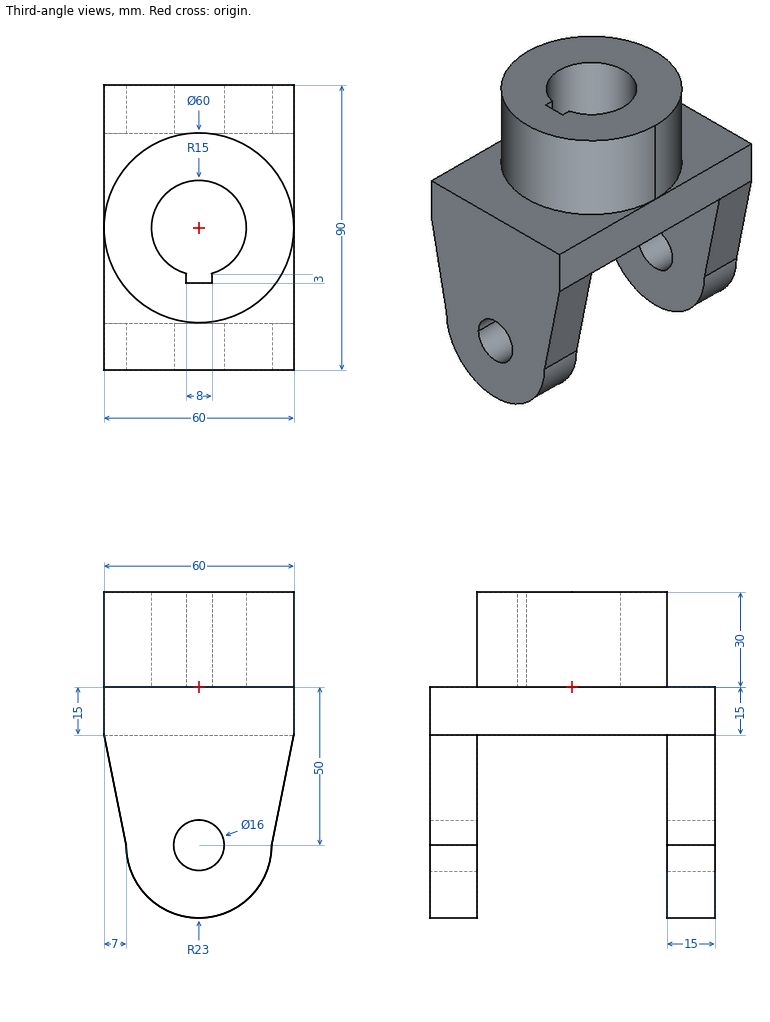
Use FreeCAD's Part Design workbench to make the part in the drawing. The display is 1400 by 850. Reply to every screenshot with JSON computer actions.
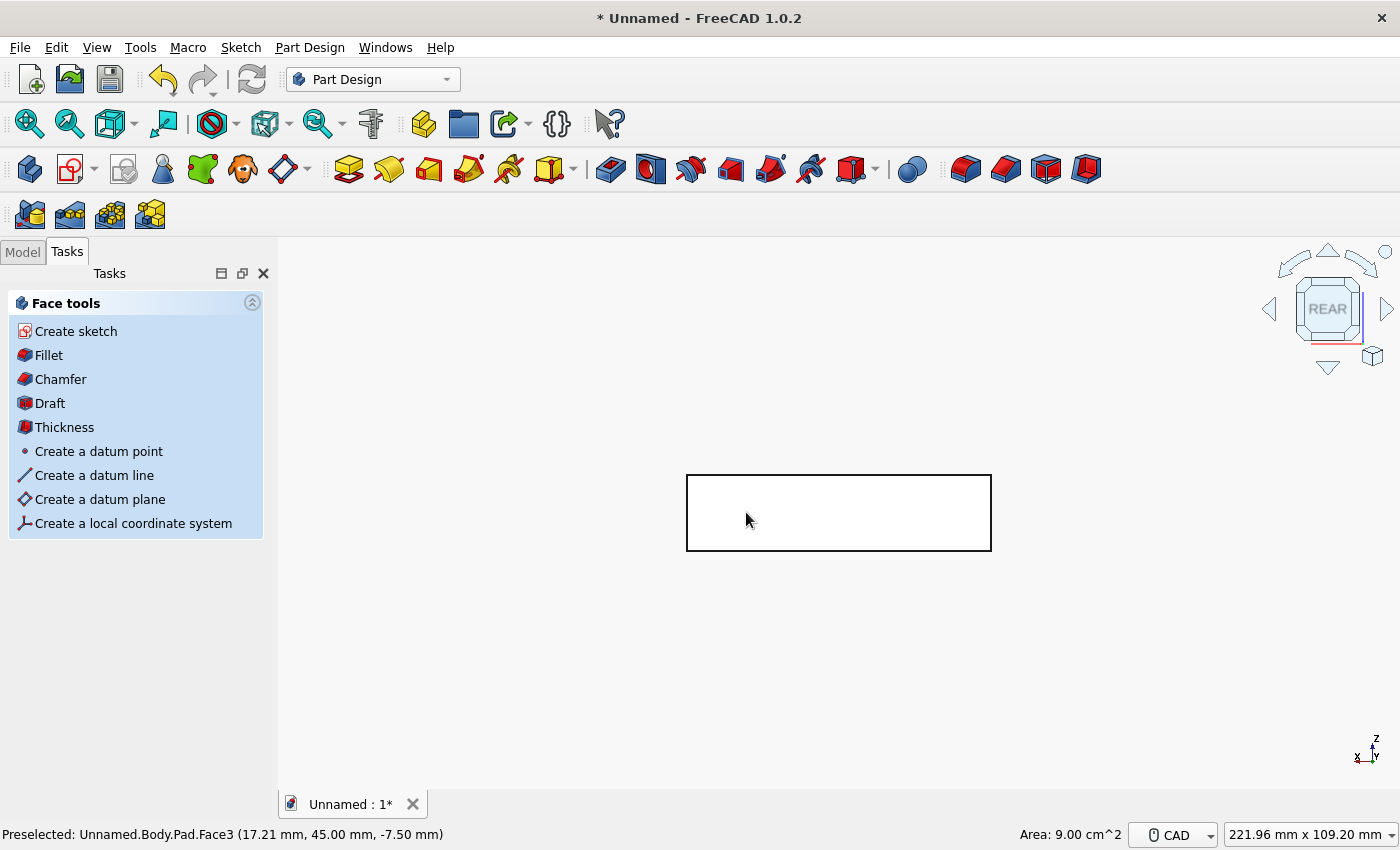
{"action": "left_click", "coordinate": [70, 170]}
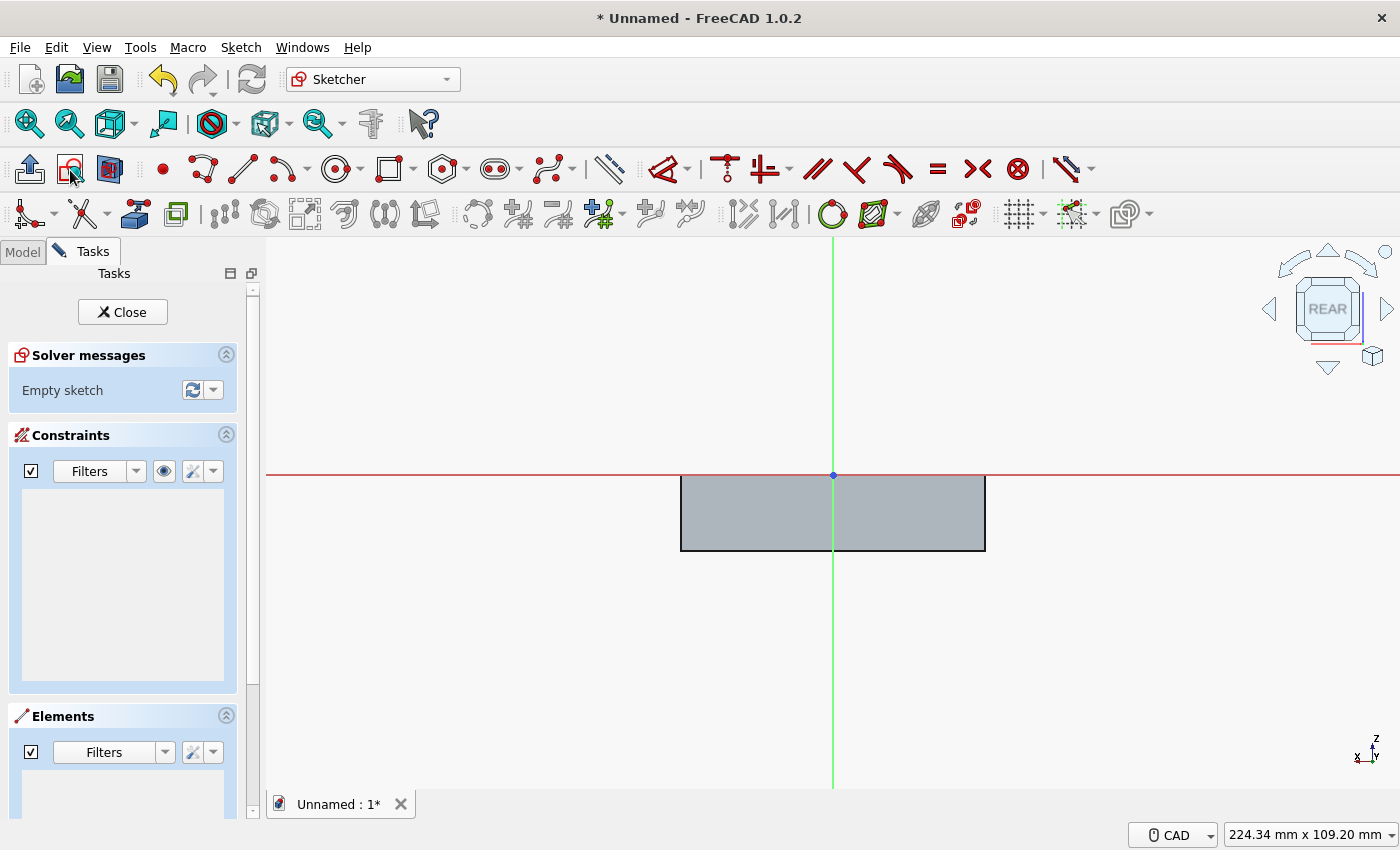
{"action": "scroll", "coordinate": [625, 265], "scroll_direction": "down", "scroll_amount": 2}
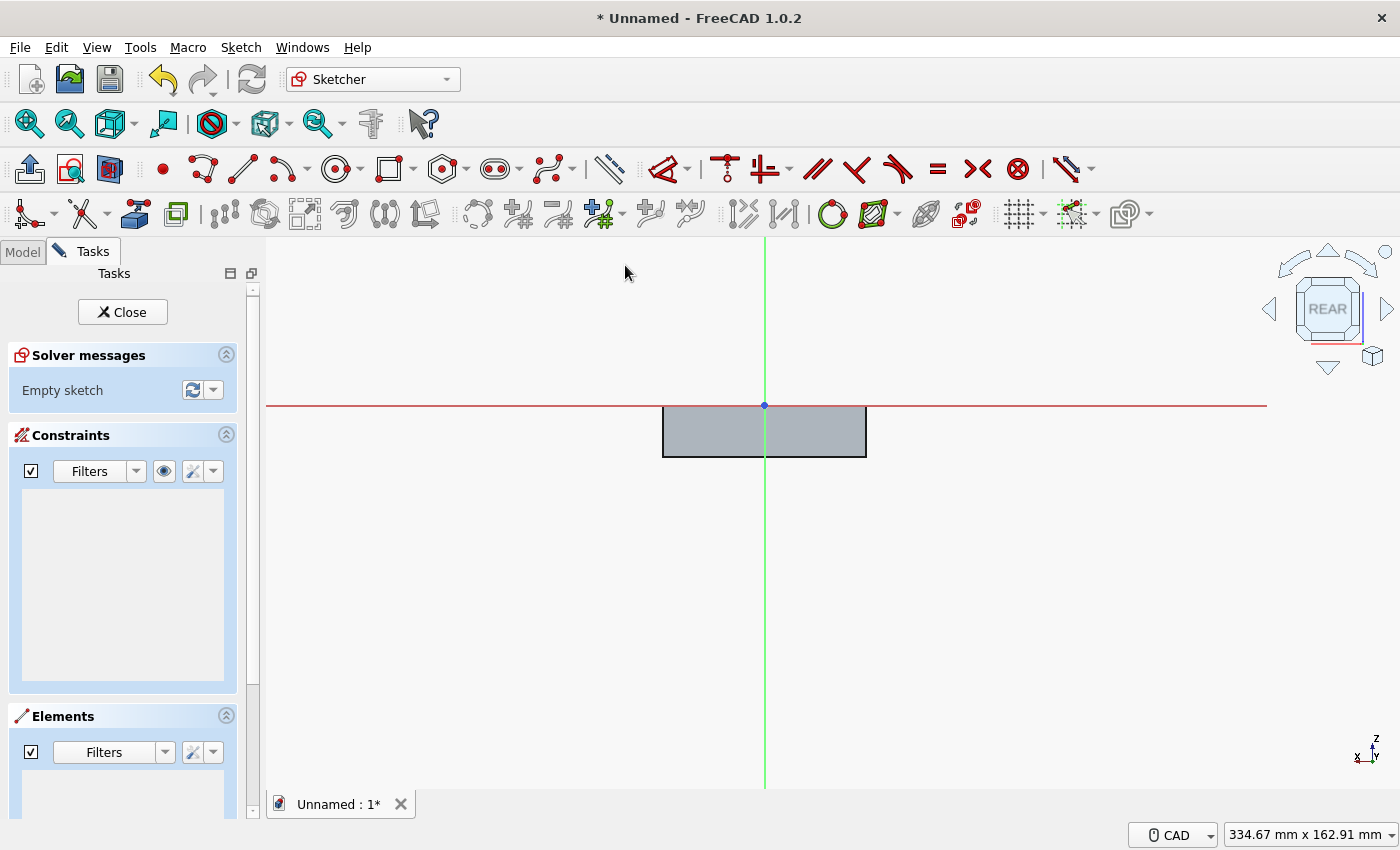
{"action": "scroll", "coordinate": [765, 563], "scroll_direction": "up", "scroll_amount": 2}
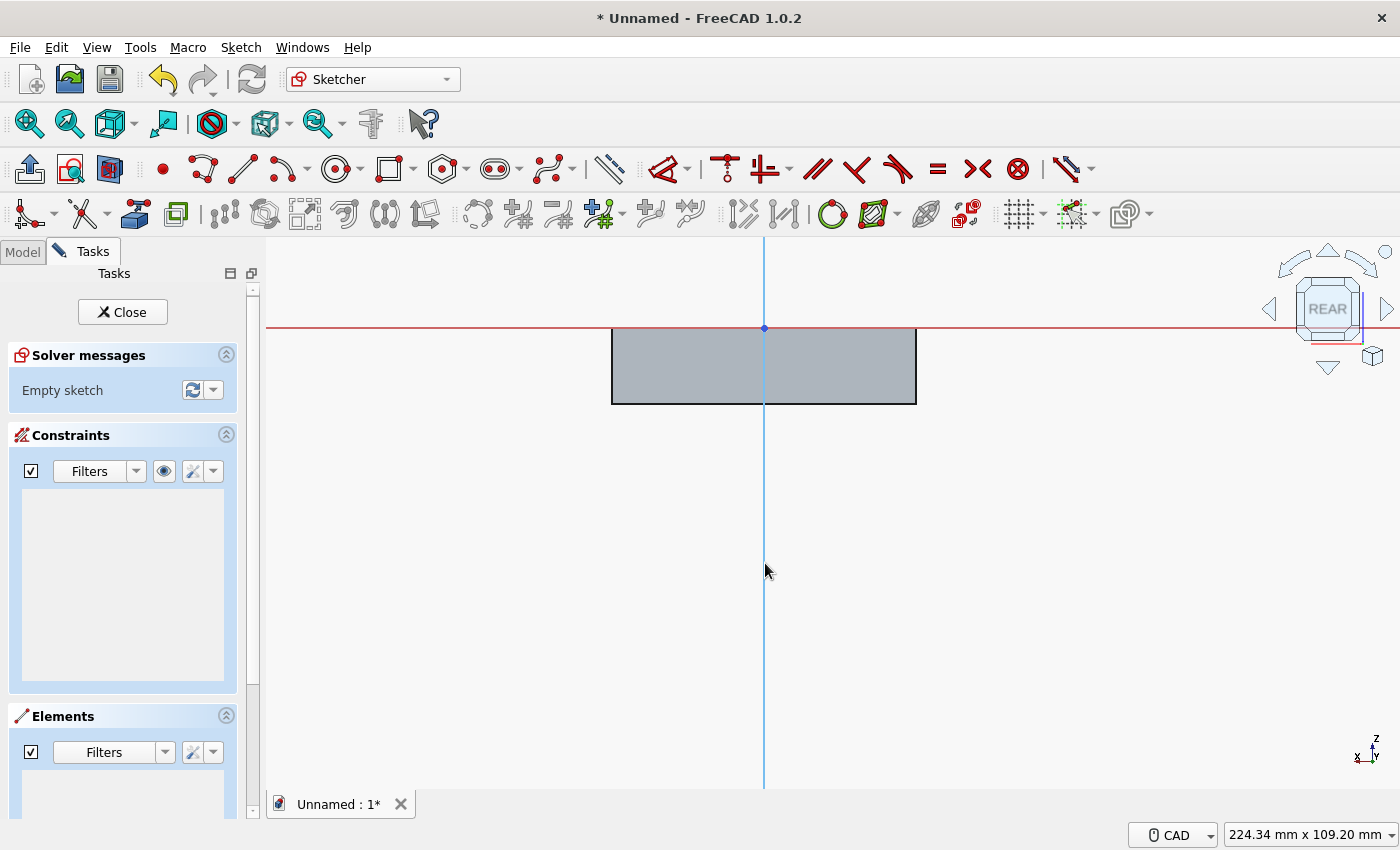
{"action": "left_click", "coordinate": [204, 170]}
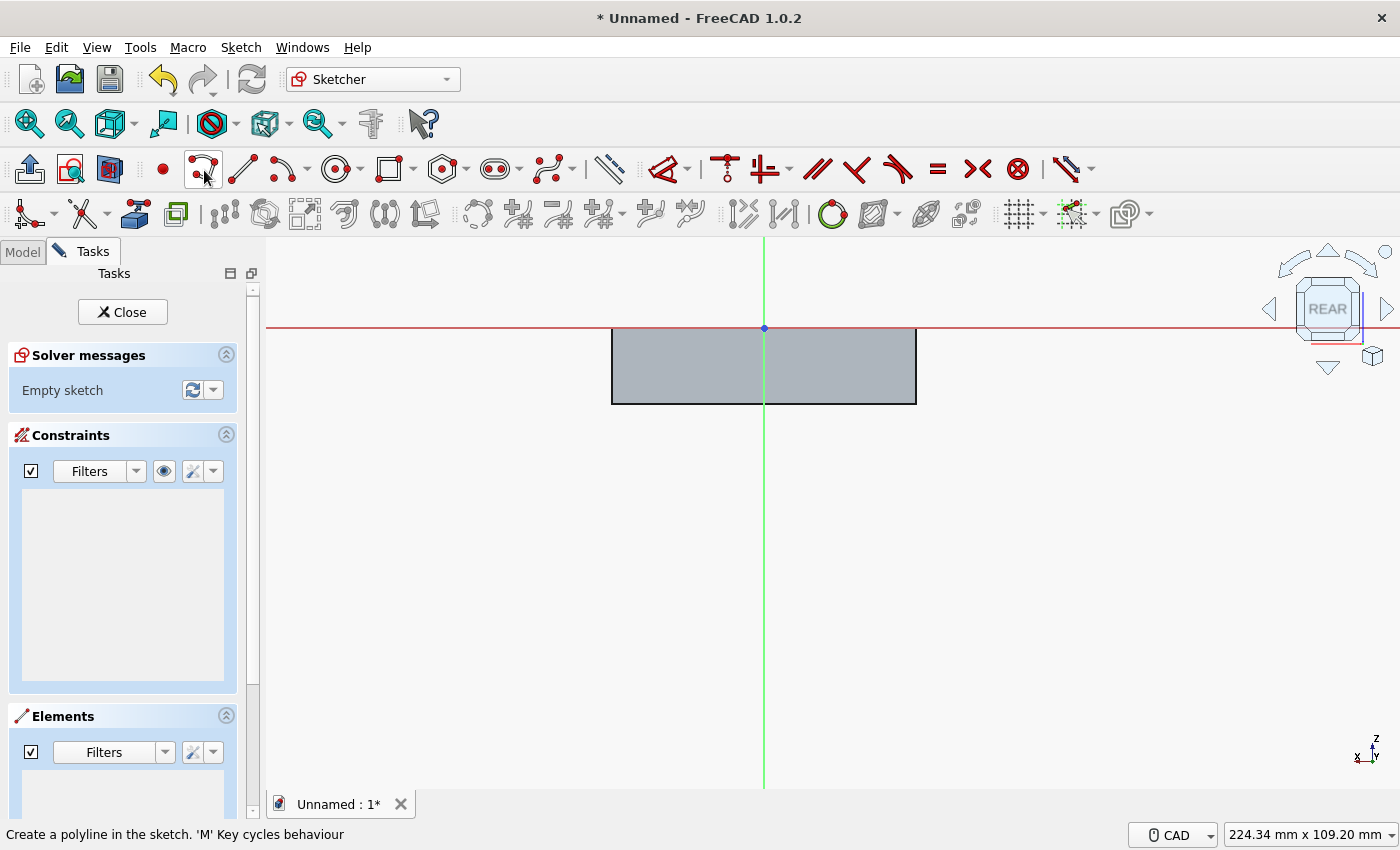
{"action": "left_click", "coordinate": [880, 581]}
{"action": "left_click", "coordinate": [916, 404]}
{"action": "left_click", "coordinate": [612, 404]}
{"action": "left_click", "coordinate": [648, 581]}
{"action": "right_click", "coordinate": [648, 581]}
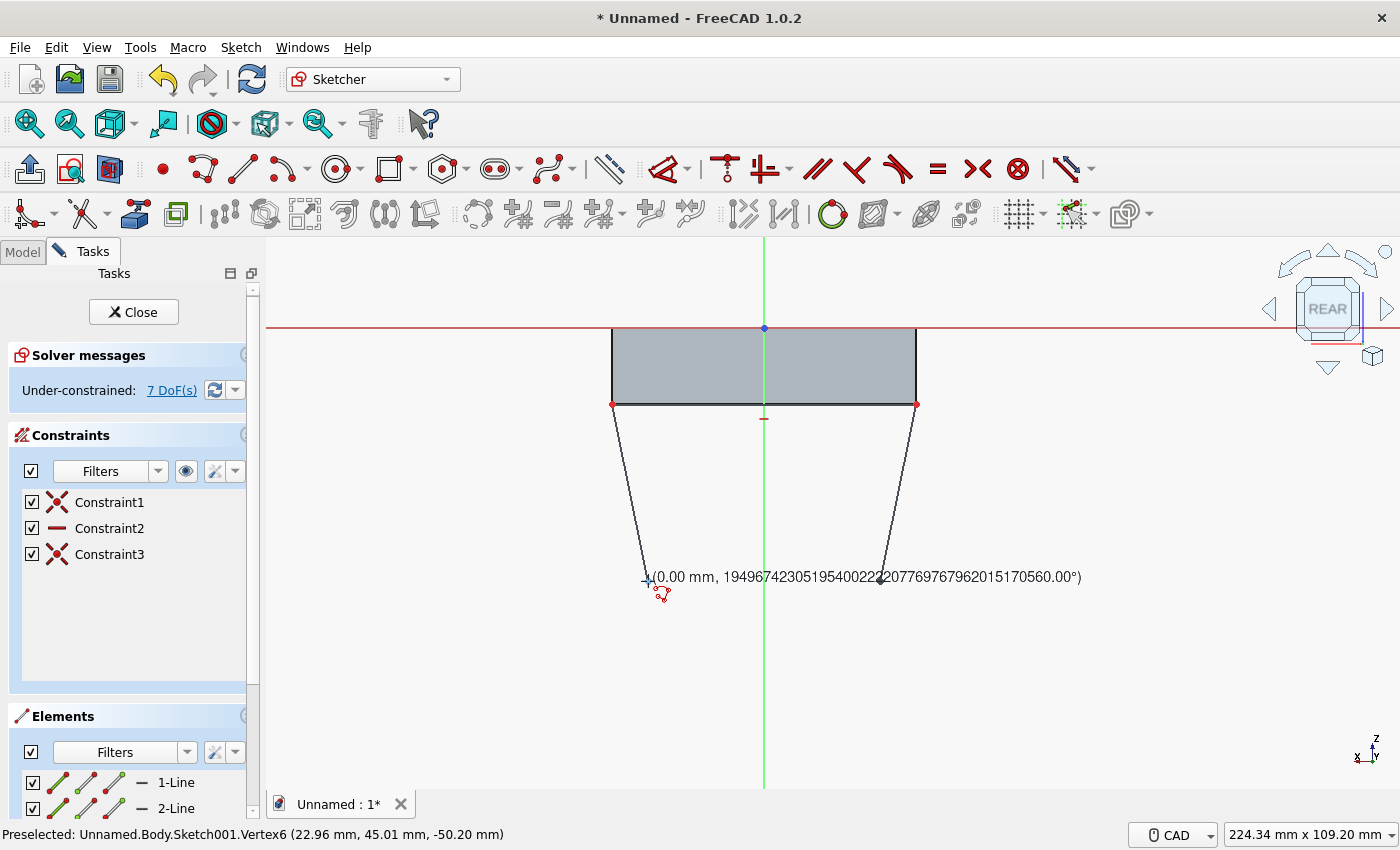
{"action": "key", "text": "g 3 a"}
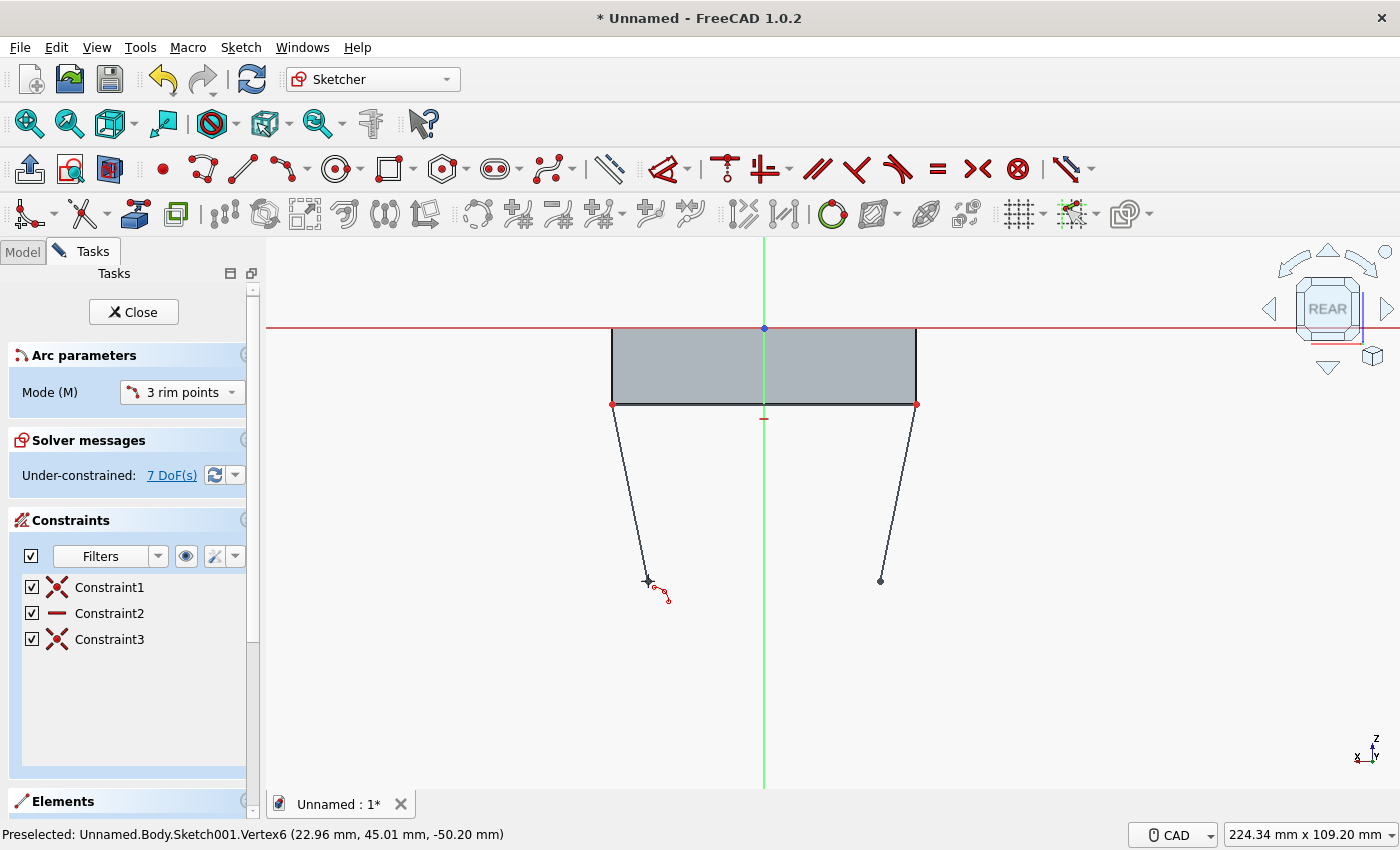
{"action": "left_click", "coordinate": [648, 582]}
{"action": "left_click", "coordinate": [880, 582]}
{"action": "left_click", "coordinate": [728, 692]}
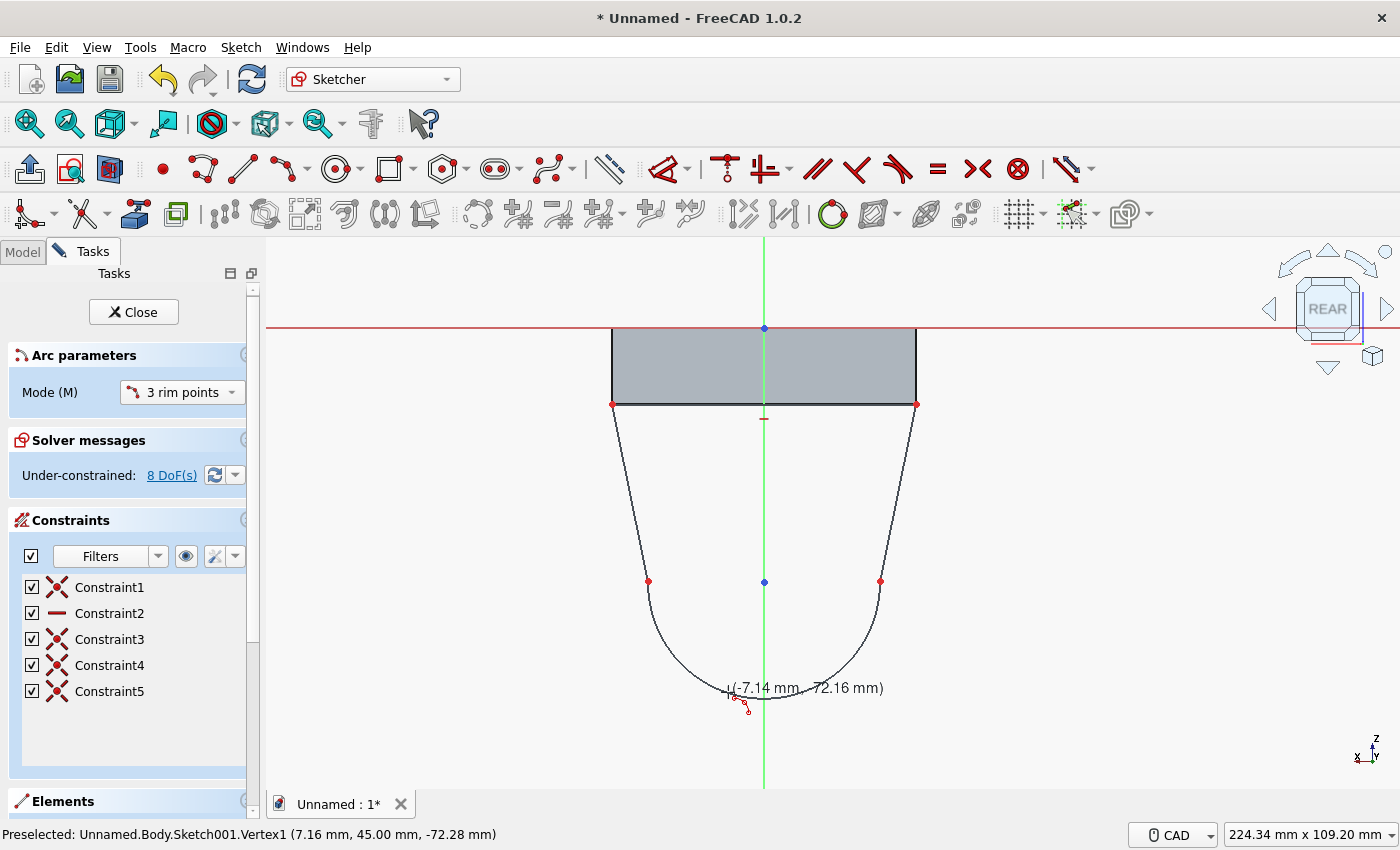
{"action": "left_click", "coordinate": [336, 170]}